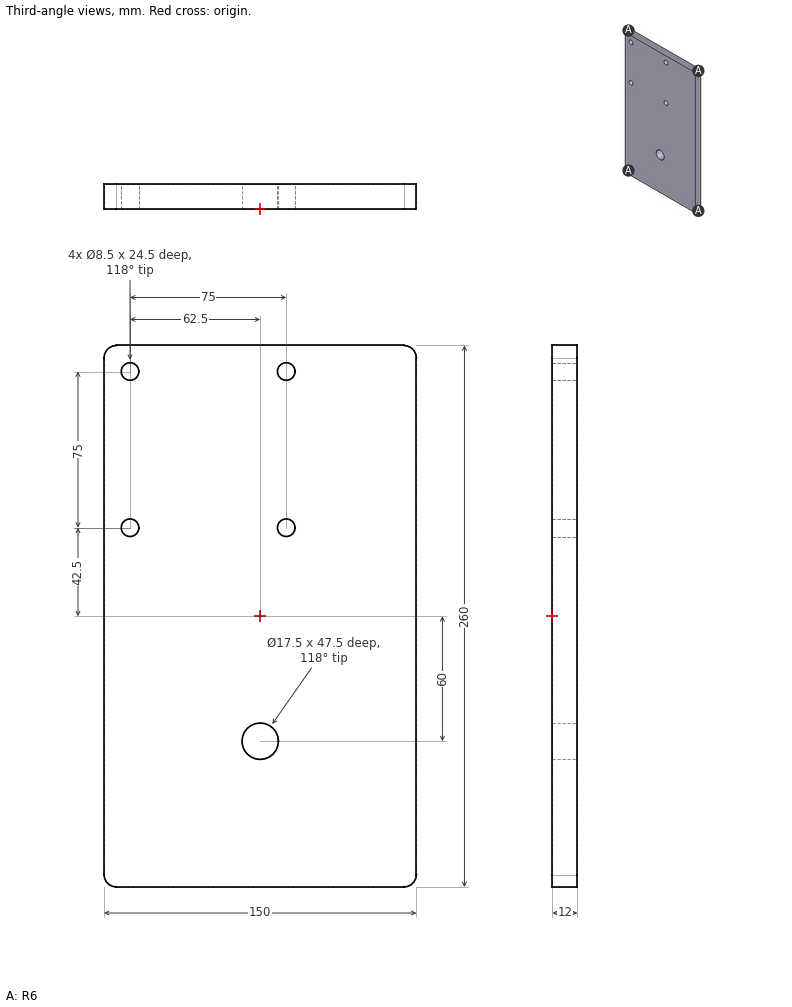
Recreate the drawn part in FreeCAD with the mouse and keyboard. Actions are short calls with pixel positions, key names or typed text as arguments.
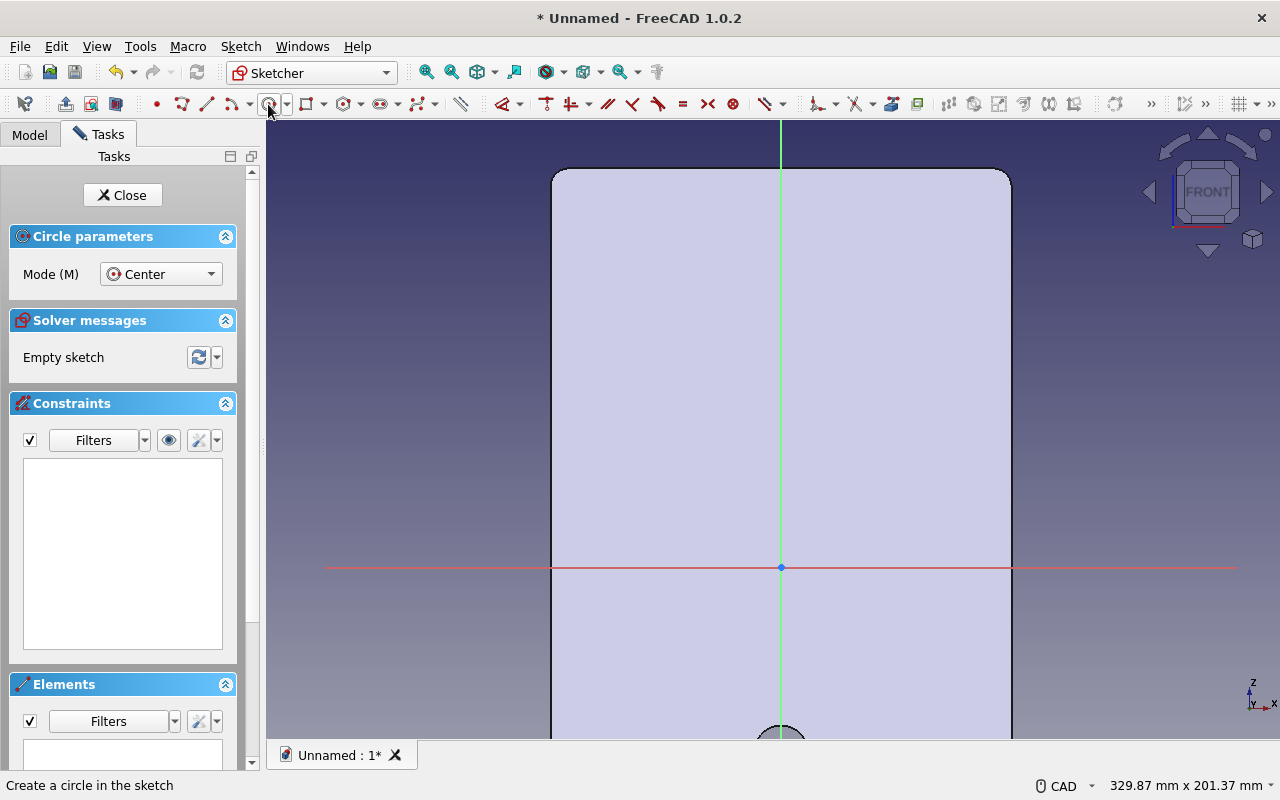
scroll(589, 207, up, 3)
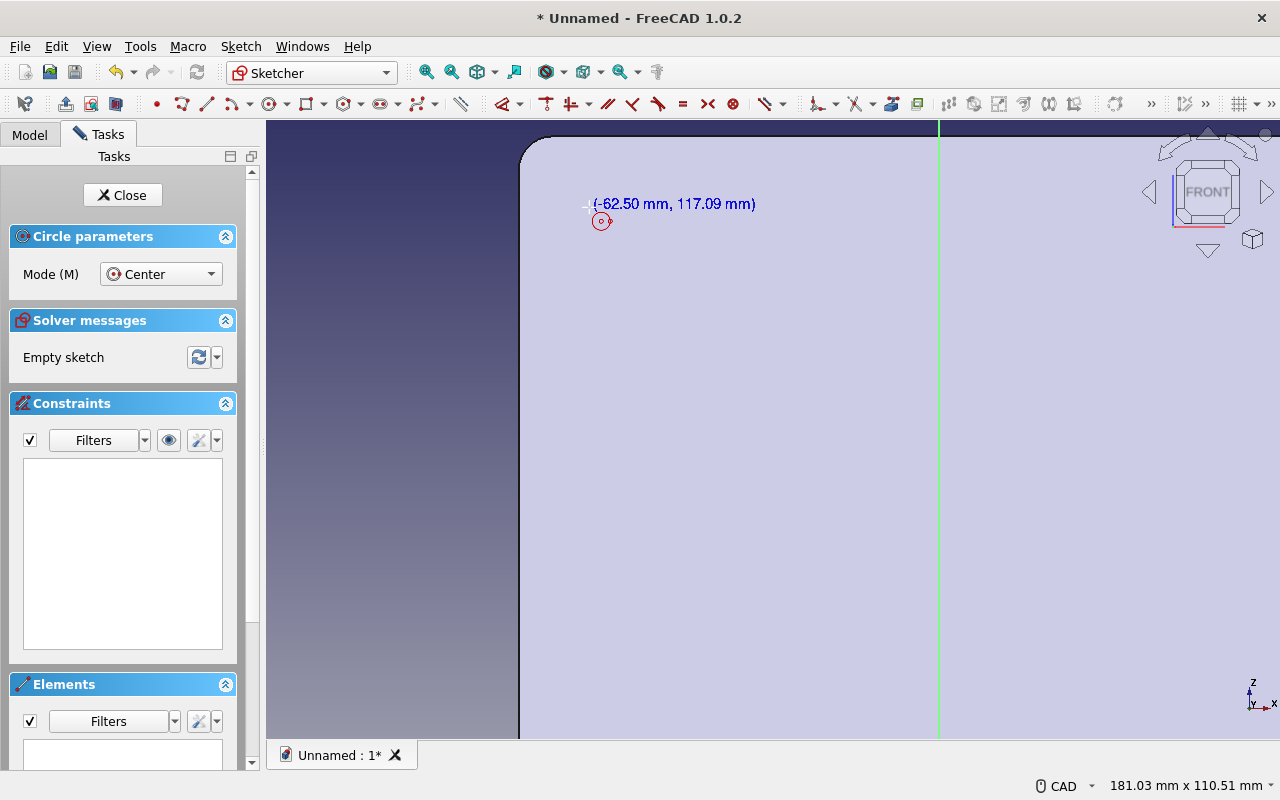
click(589, 206)
move(606, 190)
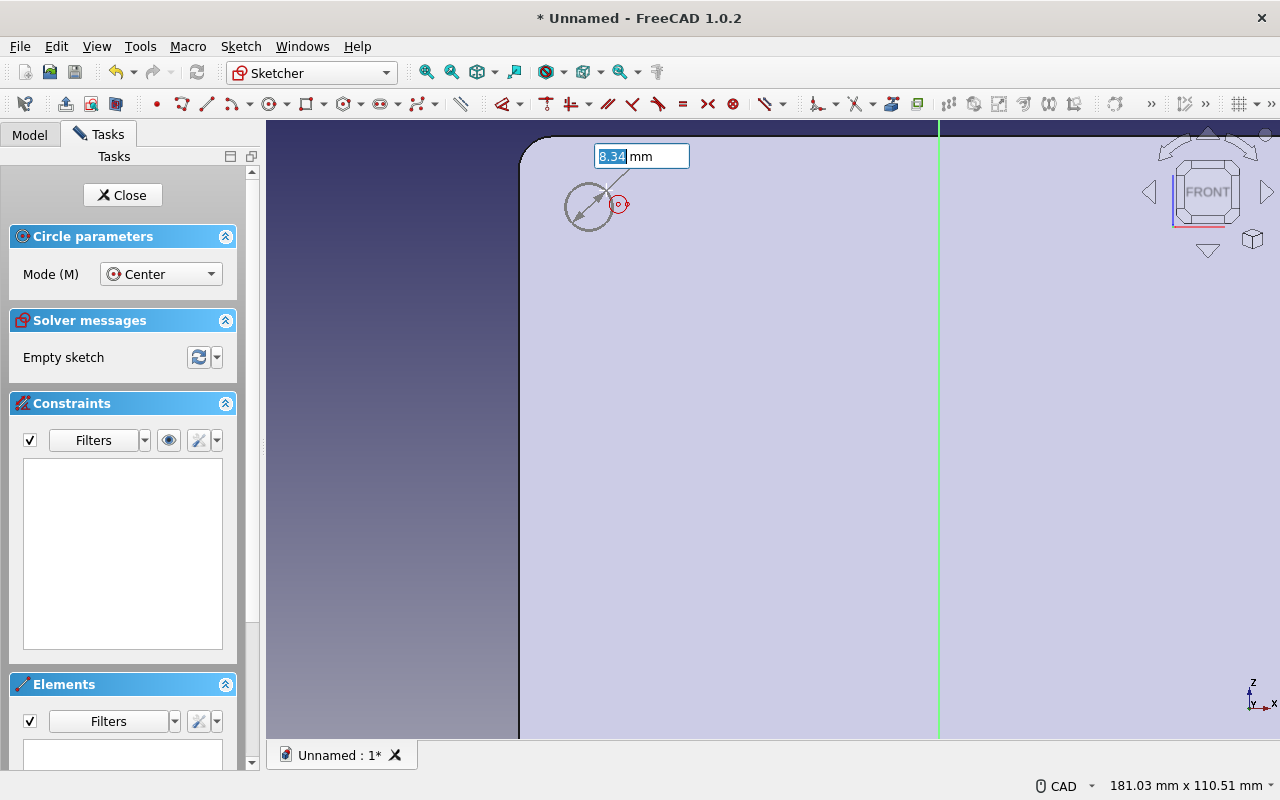
text(8.5)
key(Return)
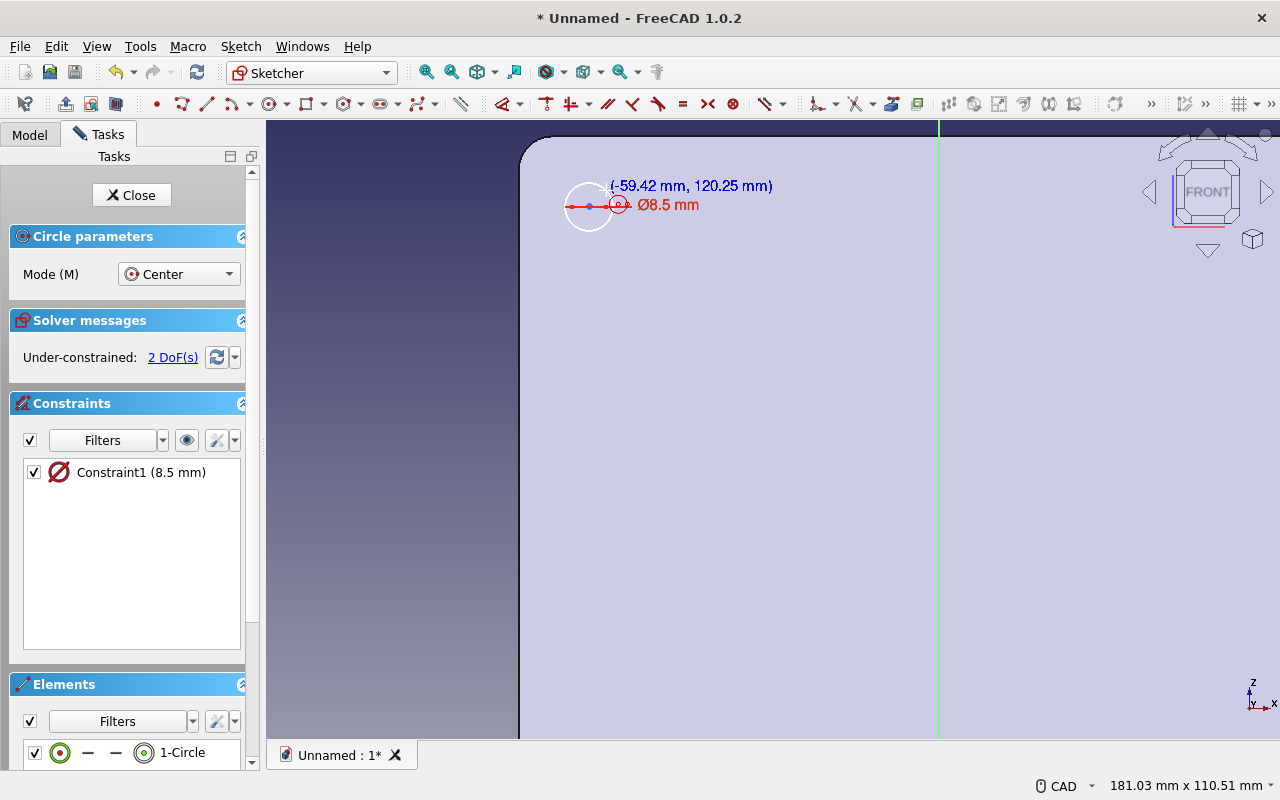
click(589, 626)
move(606, 610)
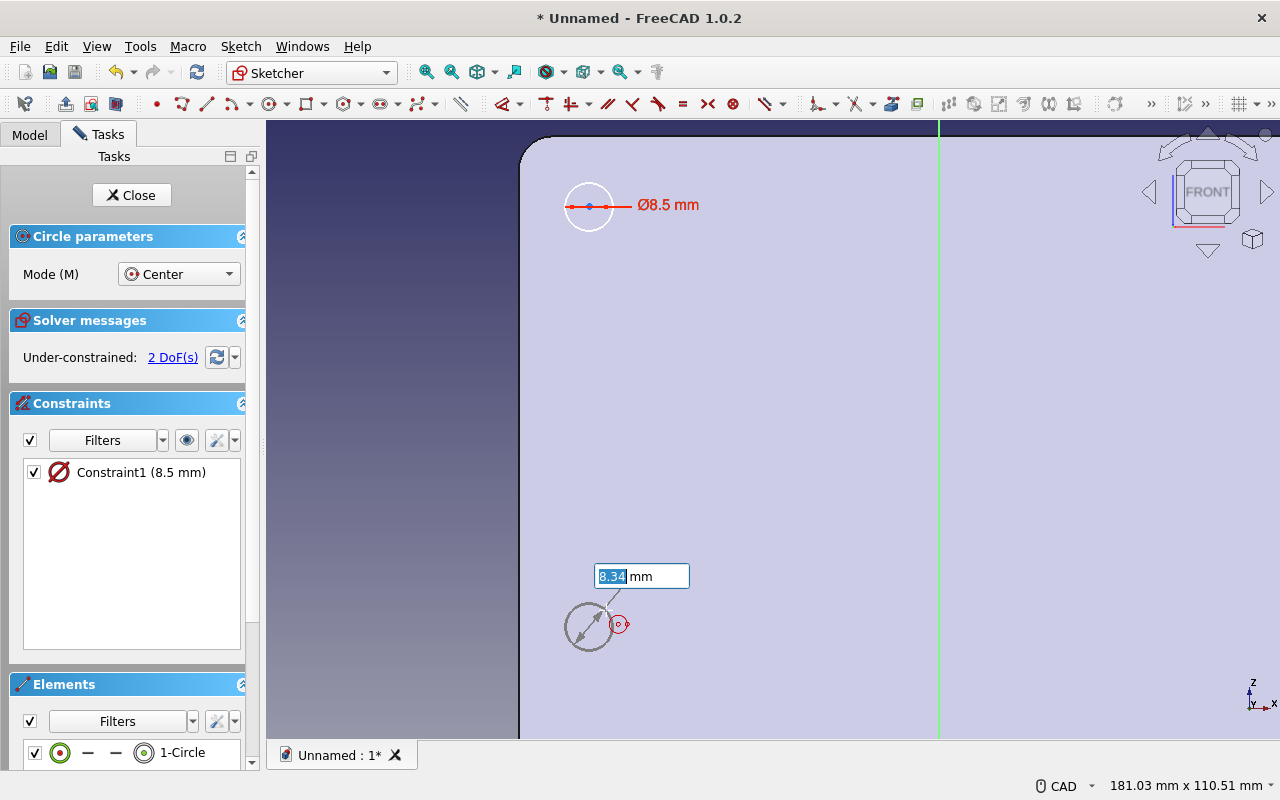
text(8.5)
key(Return)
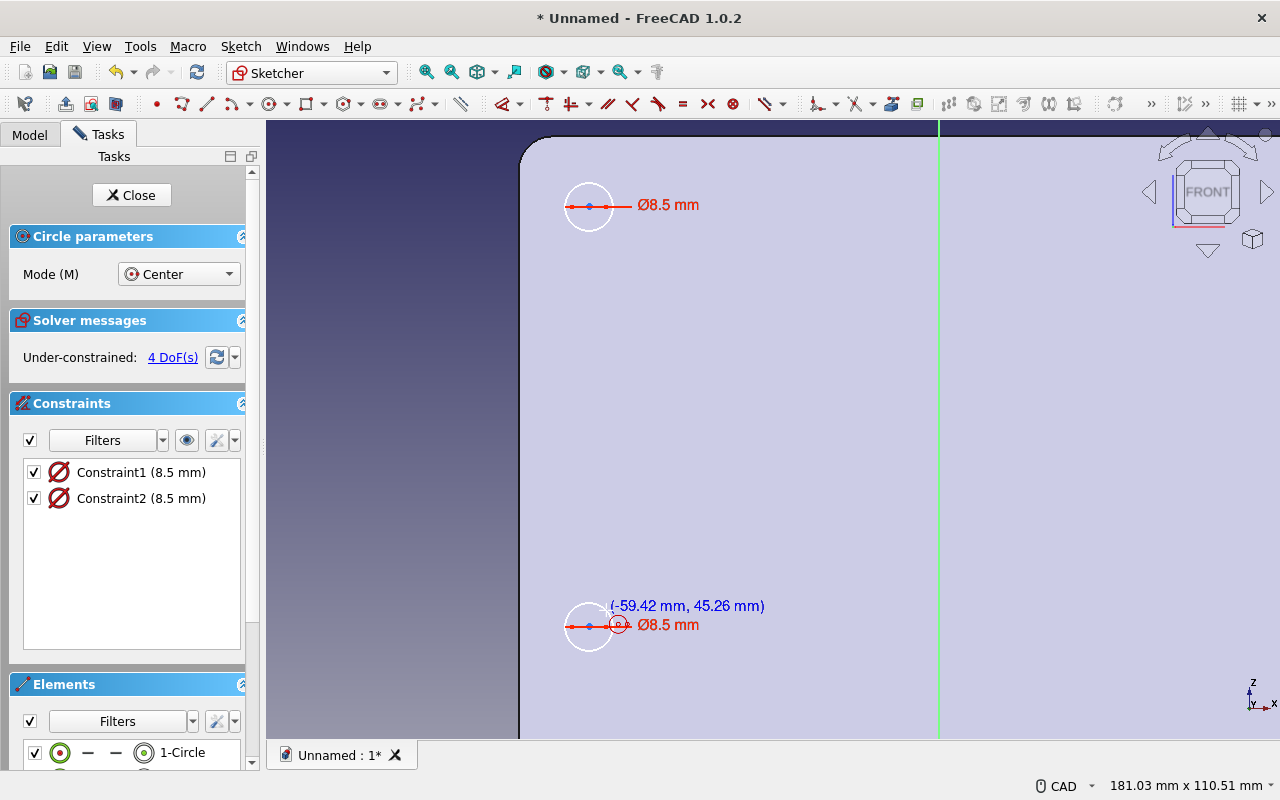
click(1009, 626)
move(1026, 610)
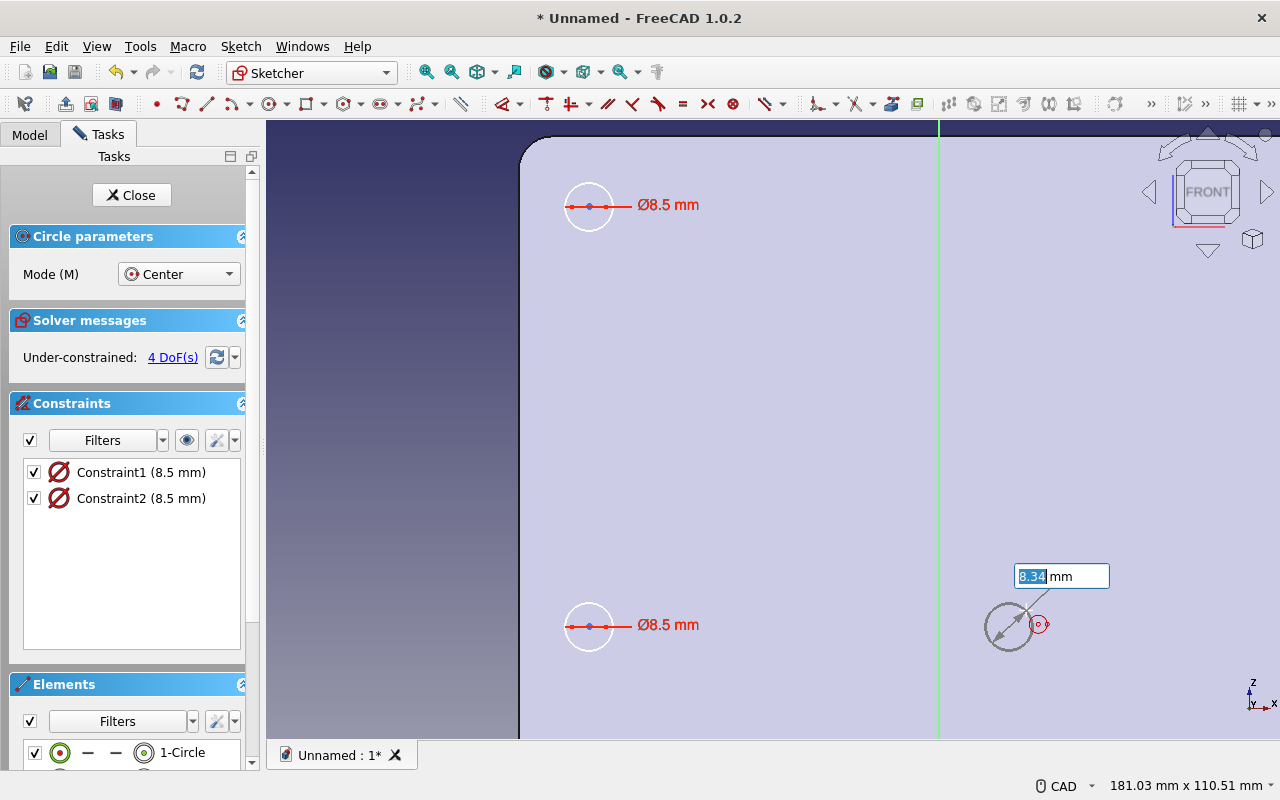
text(8.5)
key(Return)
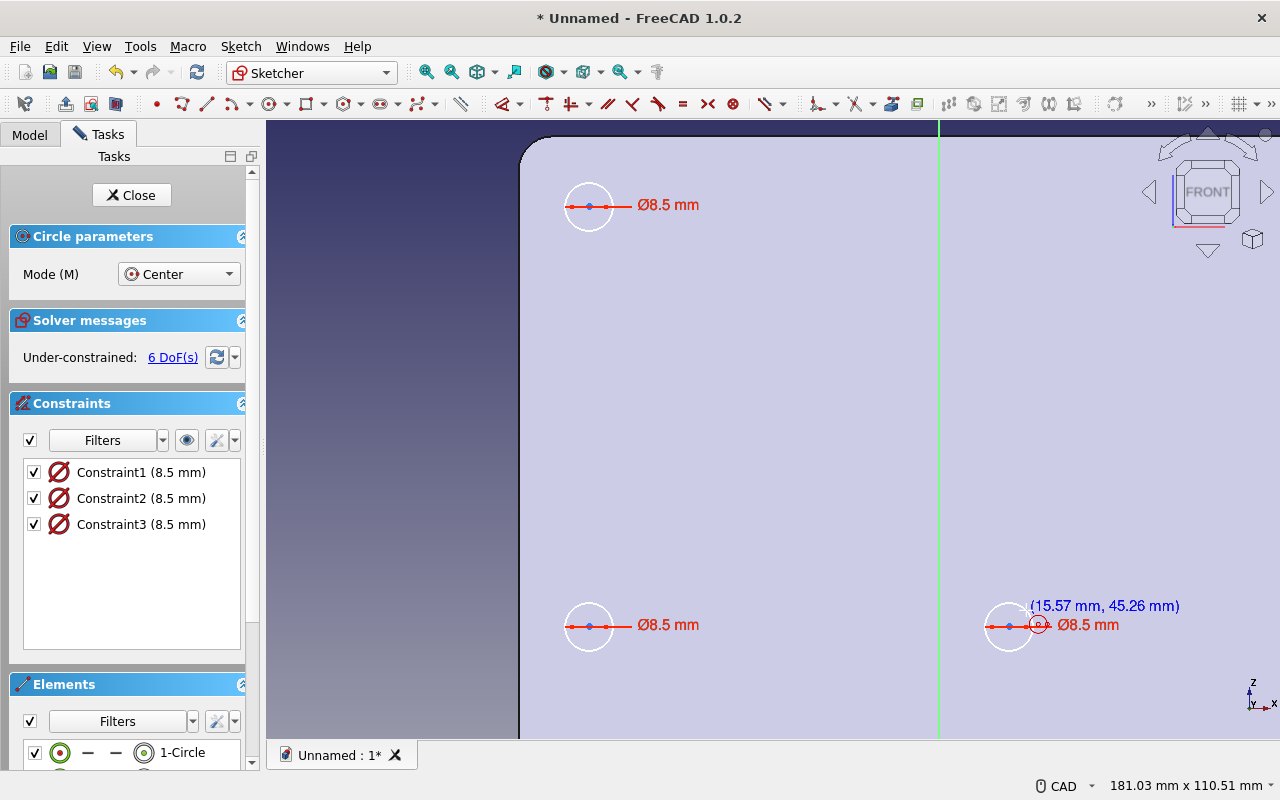
click(1009, 206)
move(1026, 190)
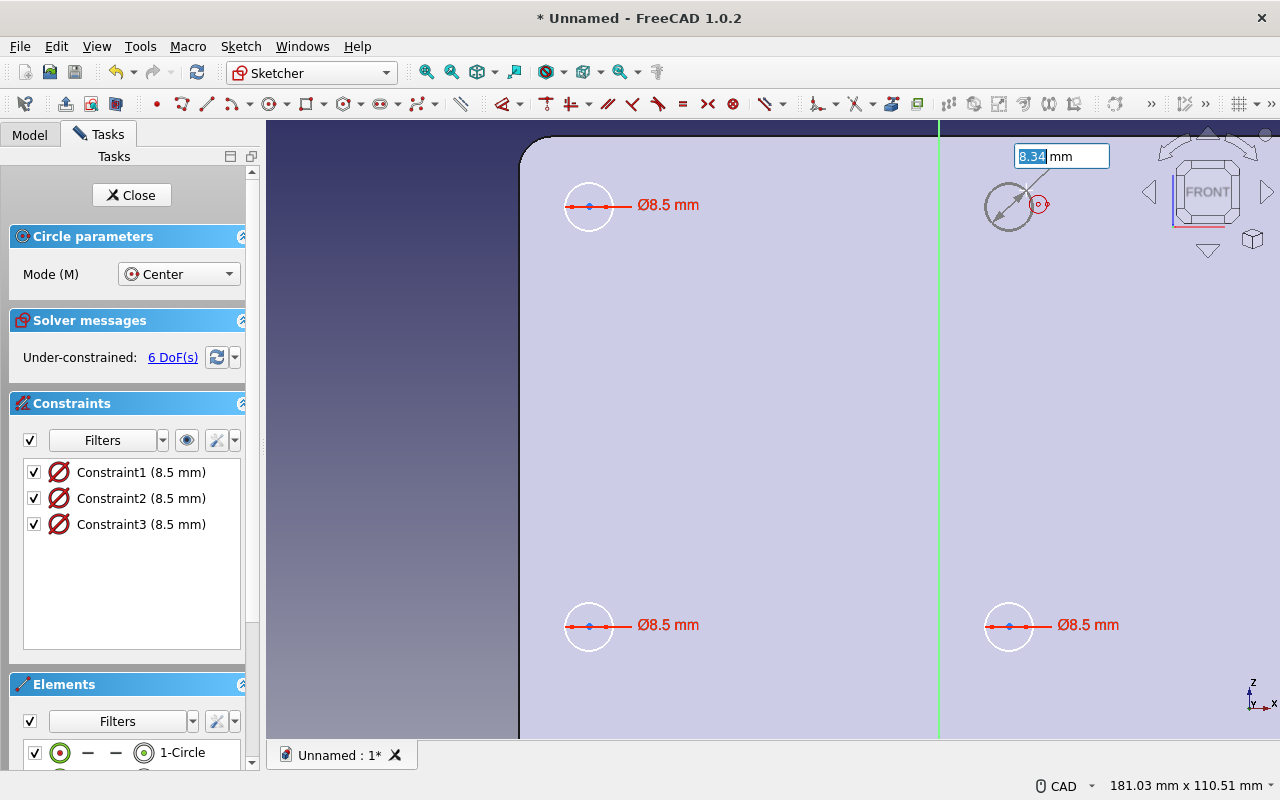
text(8.5)
key(Return)
key(Escape)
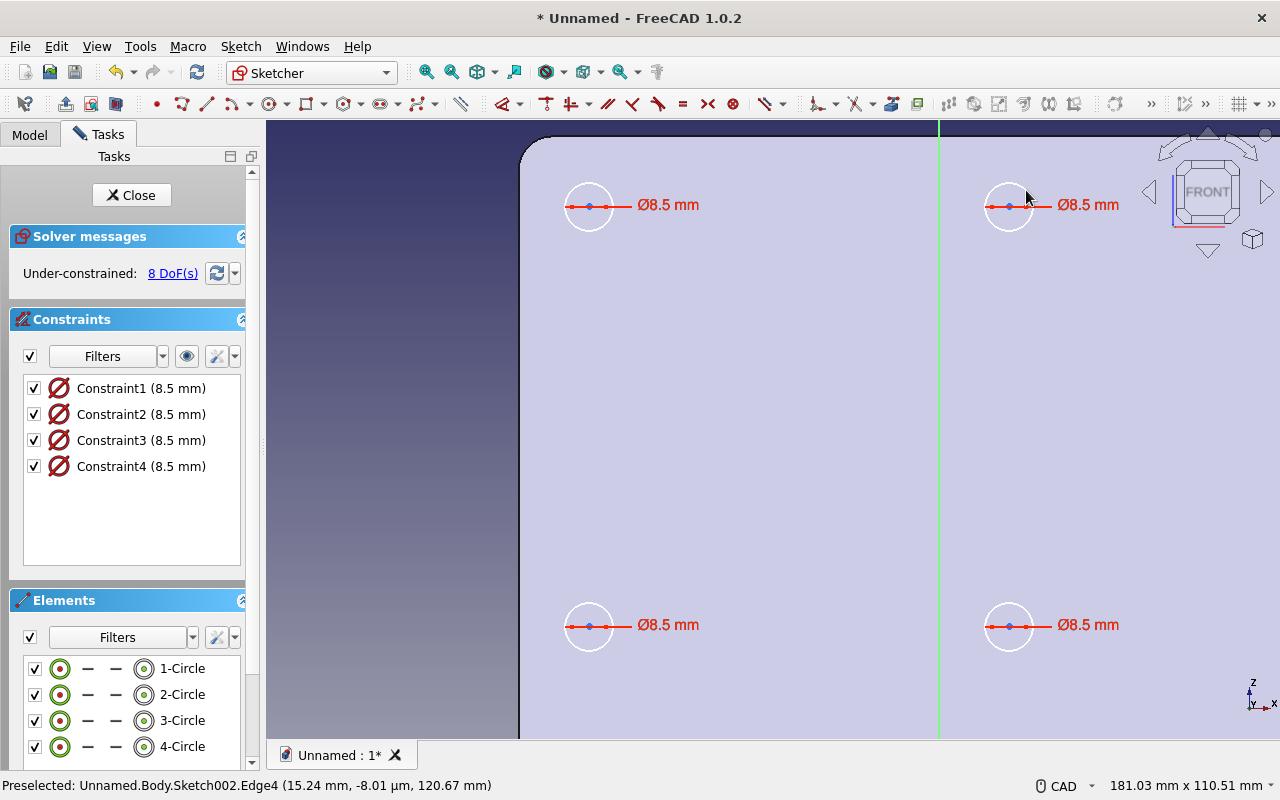
click(589, 207)